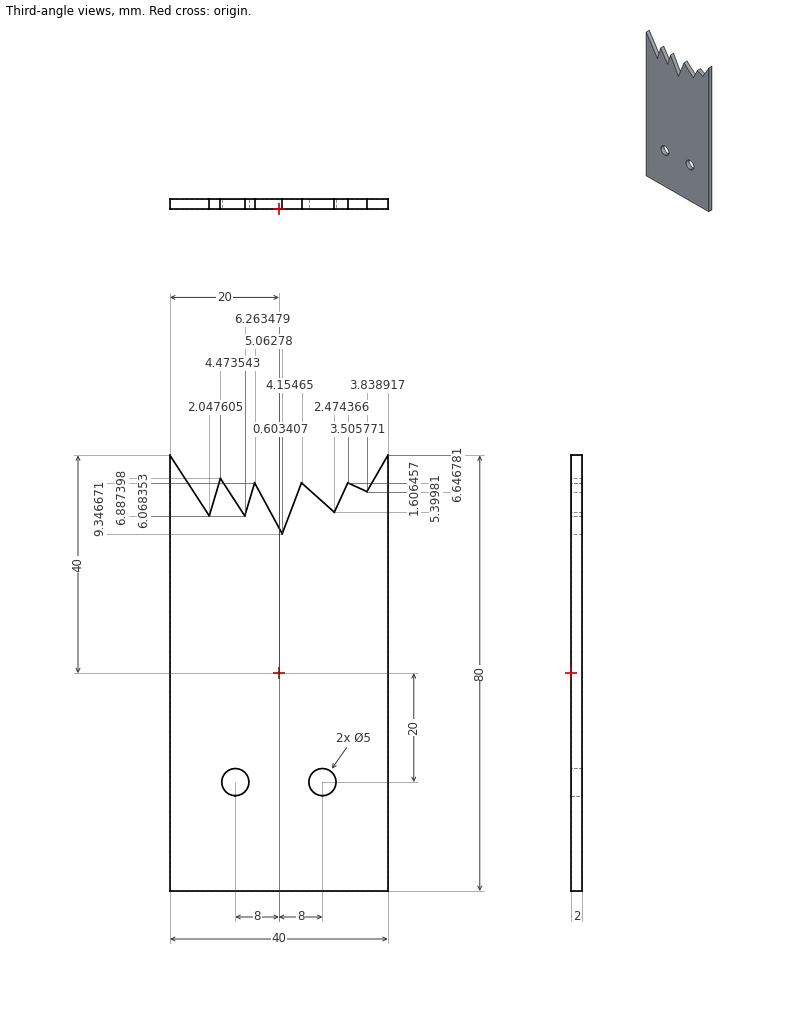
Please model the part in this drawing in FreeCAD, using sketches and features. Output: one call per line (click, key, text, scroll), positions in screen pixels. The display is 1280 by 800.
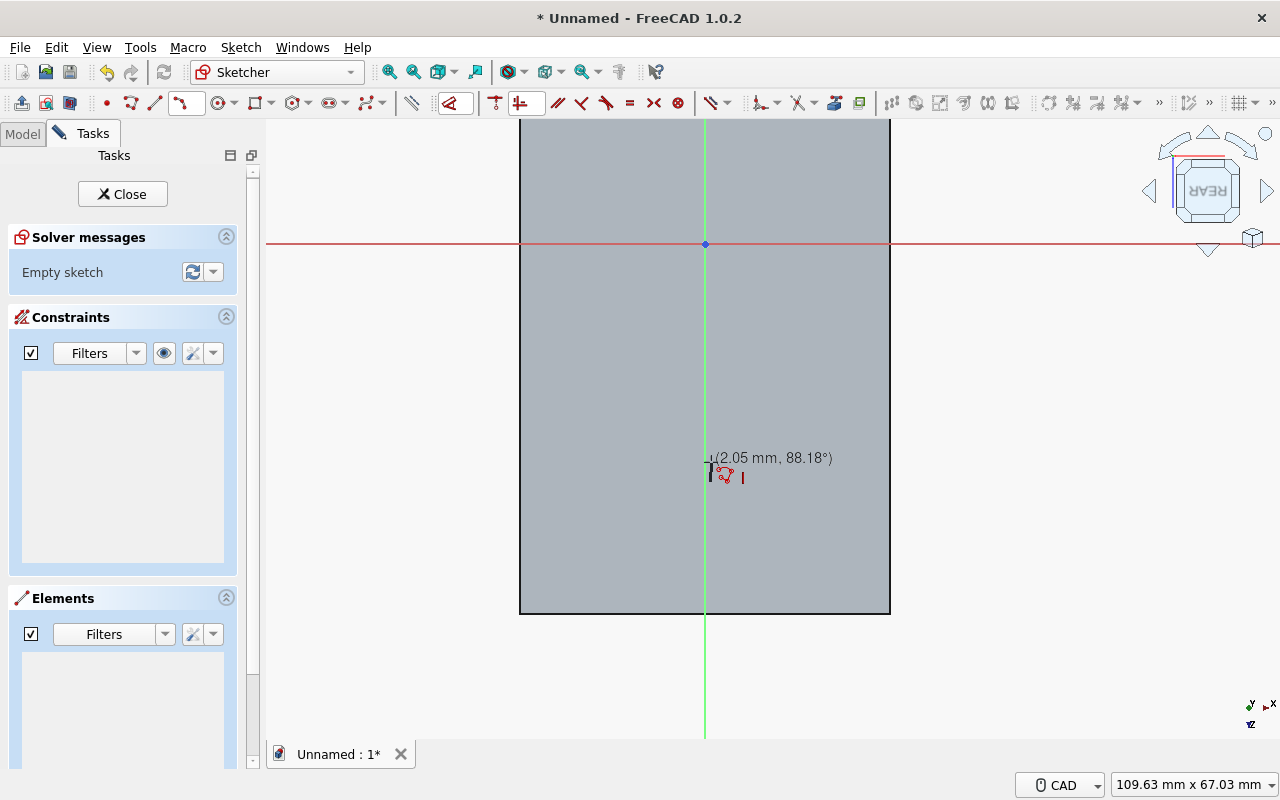
click(664, 568)
click(647, 512)
click(606, 575)
click(587, 512)
click(520, 614)
click(890, 614)
click(855, 553)
click(822, 568)
click(799, 518)
click(743, 568)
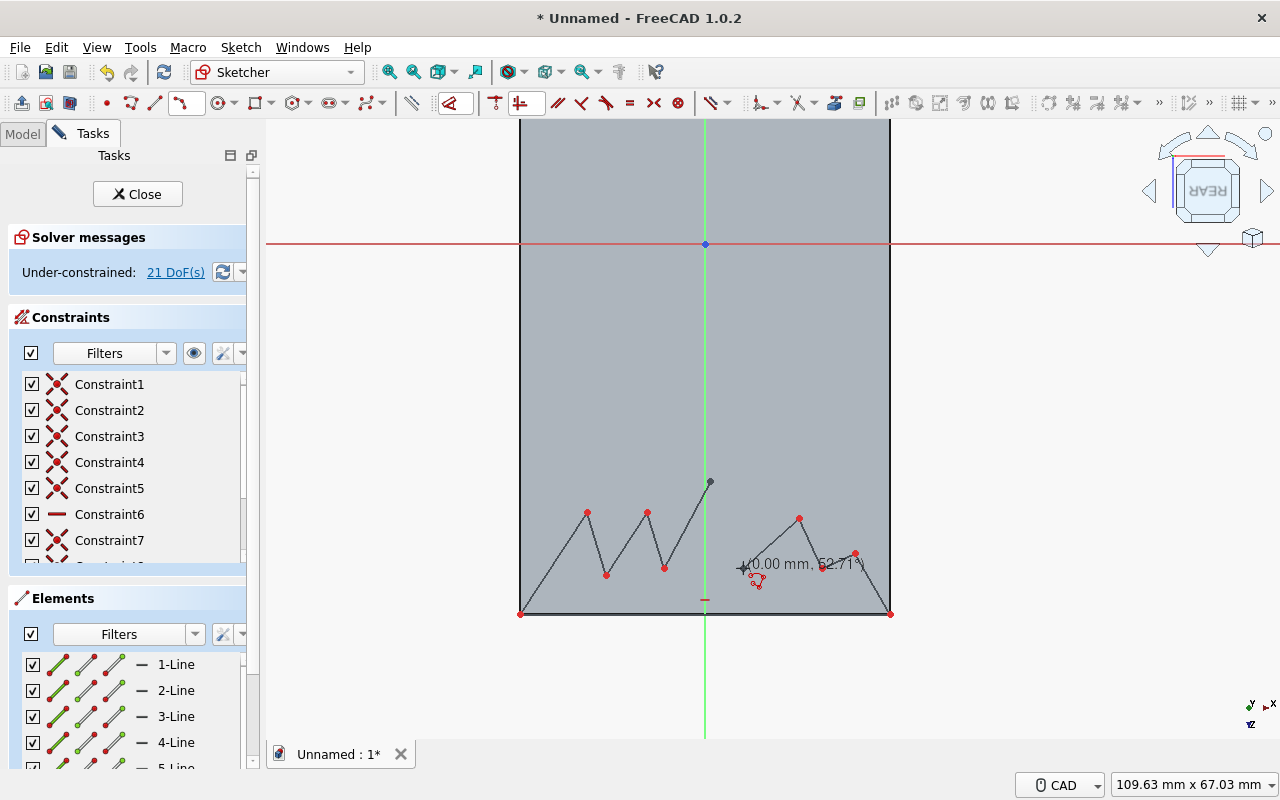
scroll(711, 481, up, 6)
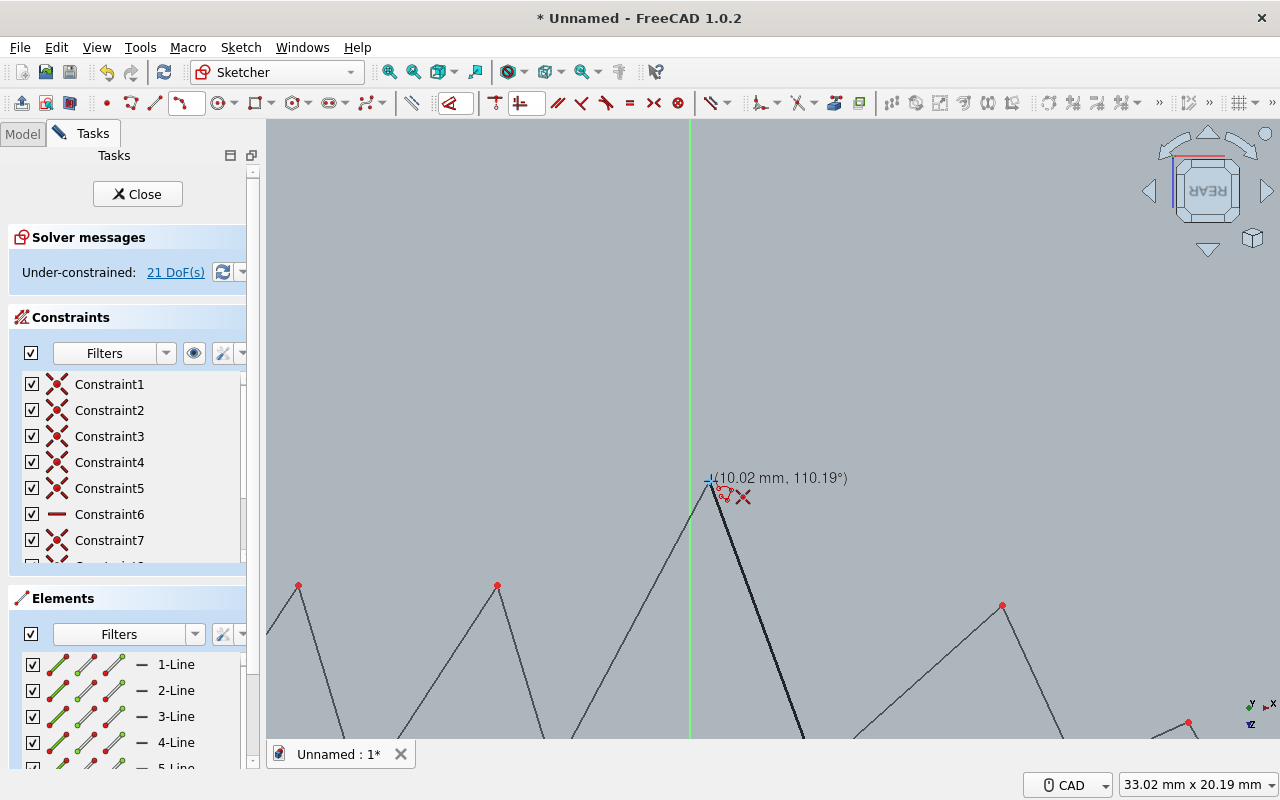
click(709, 482)
key(Escape)
key(Escape)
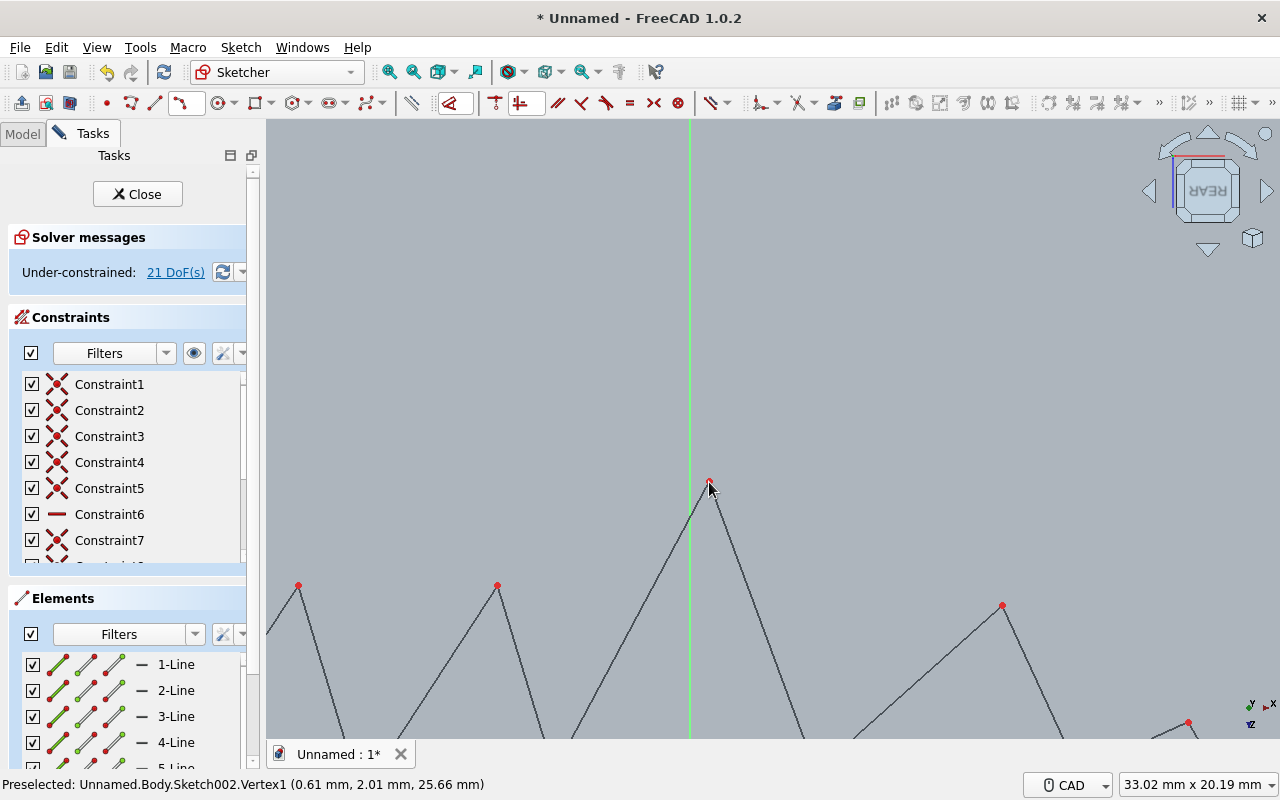
key(d)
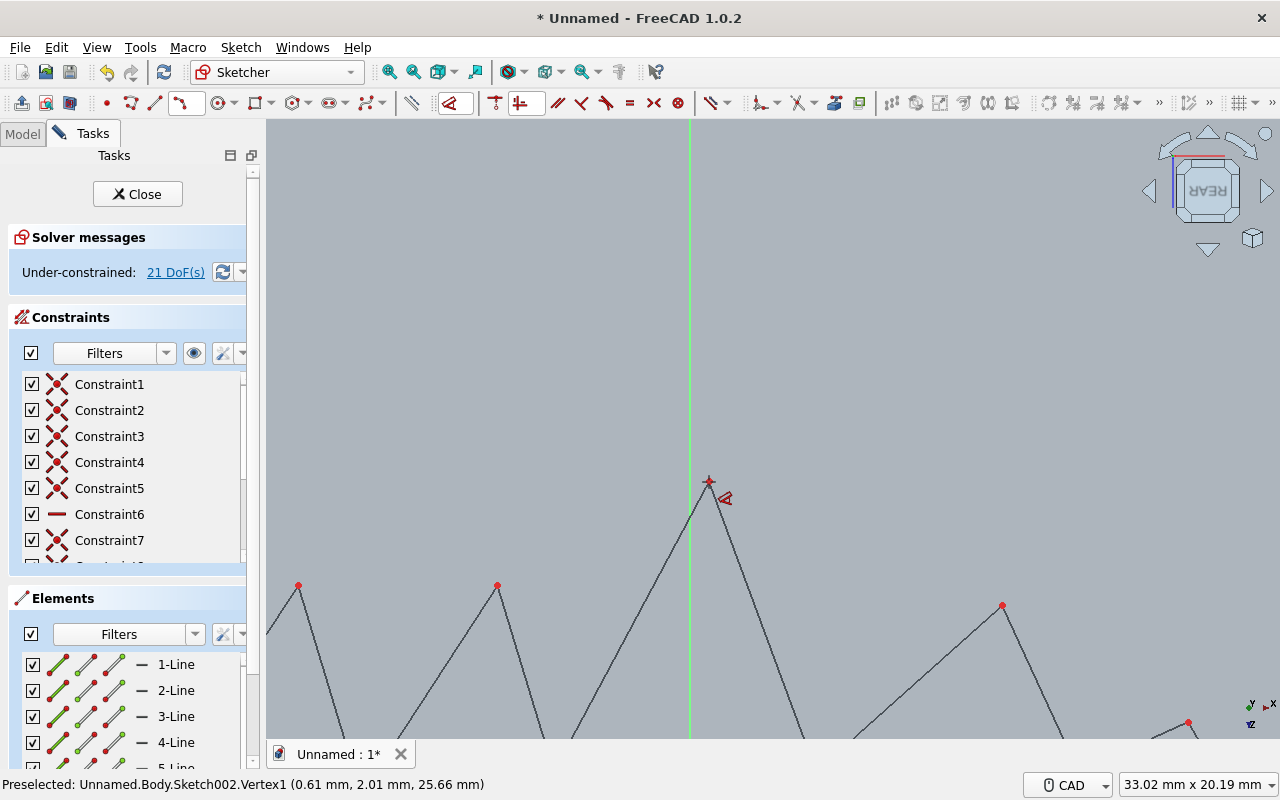
scroll(711, 481, down, 6)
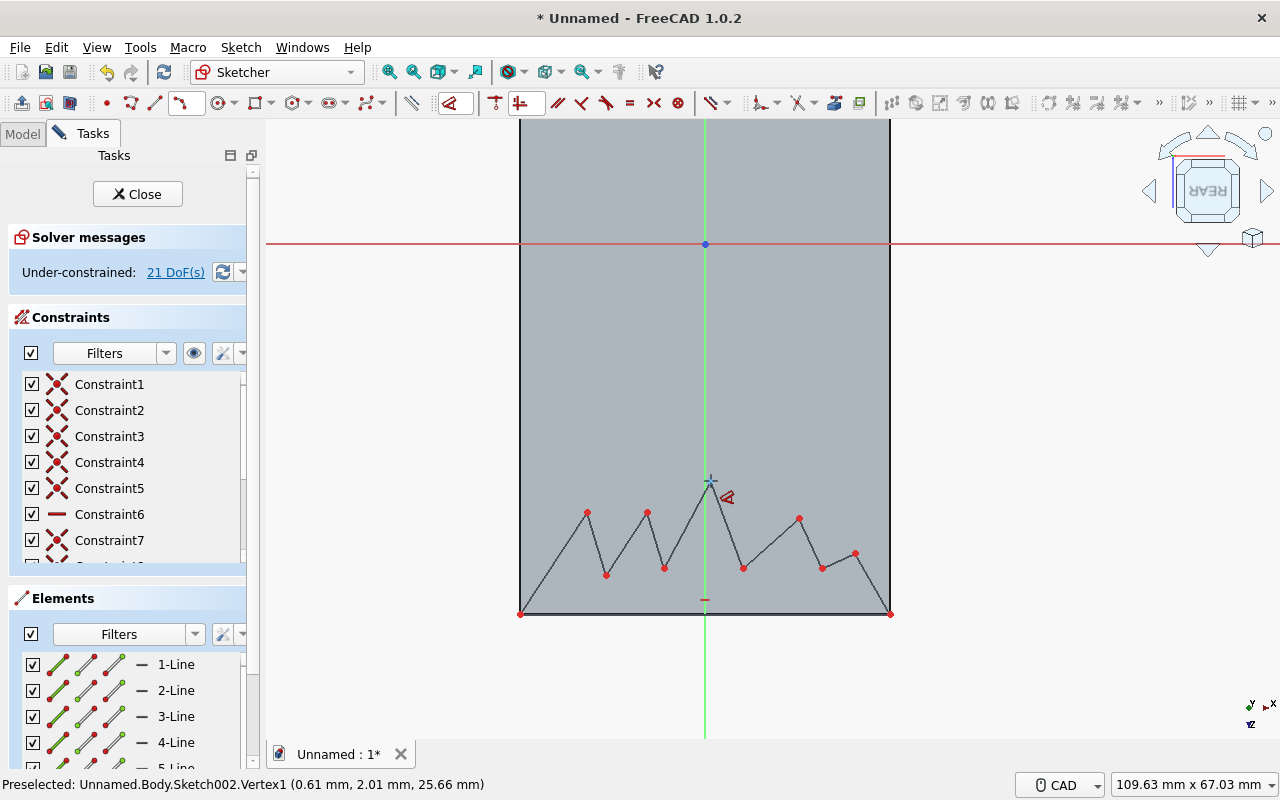
click(631, 615)
click(620, 649)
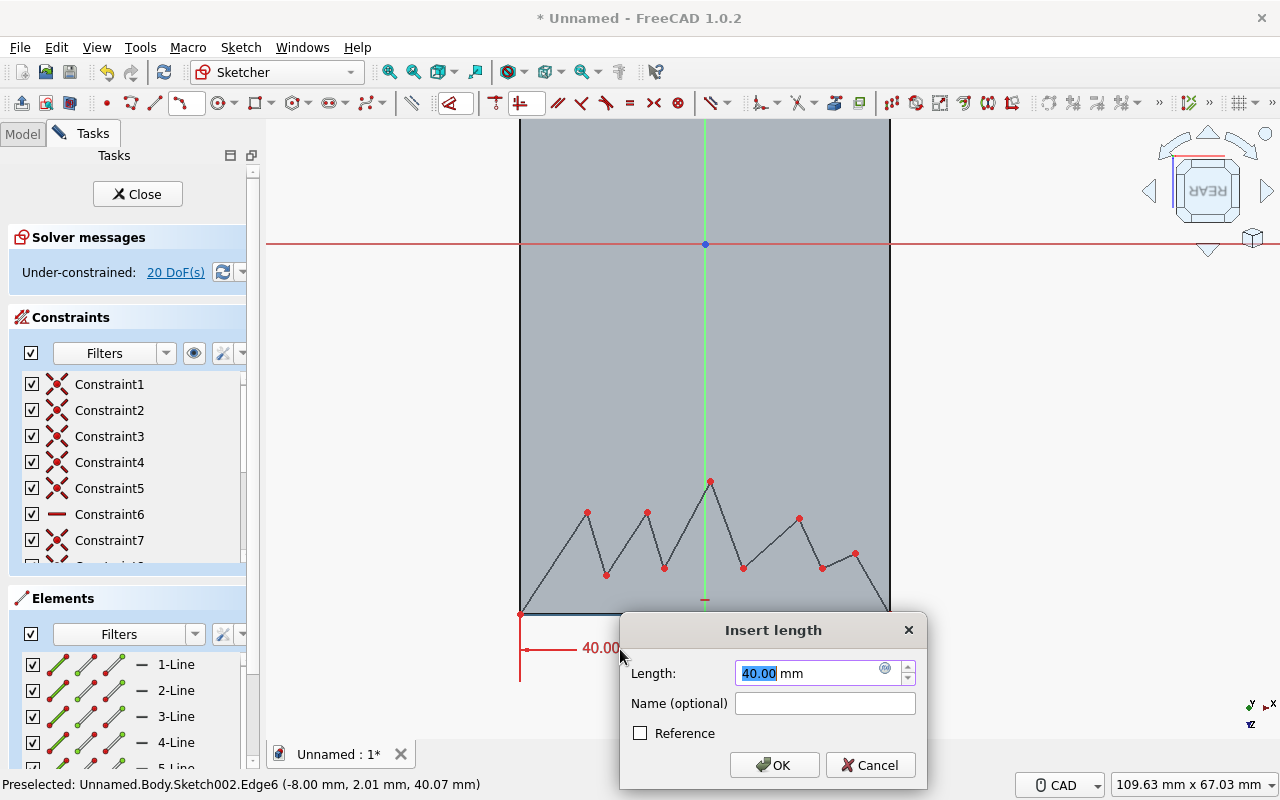
text(40)
key(Return)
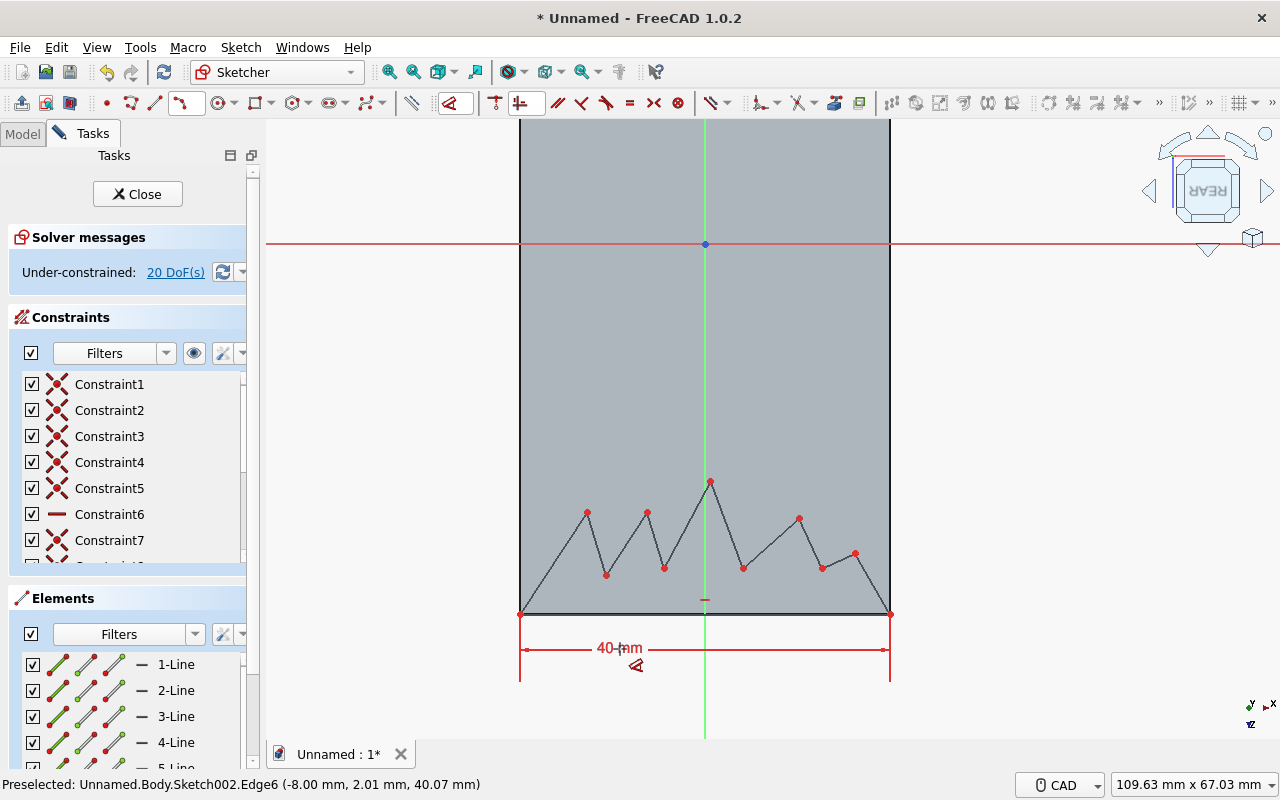
click(520, 615)
click(548, 649)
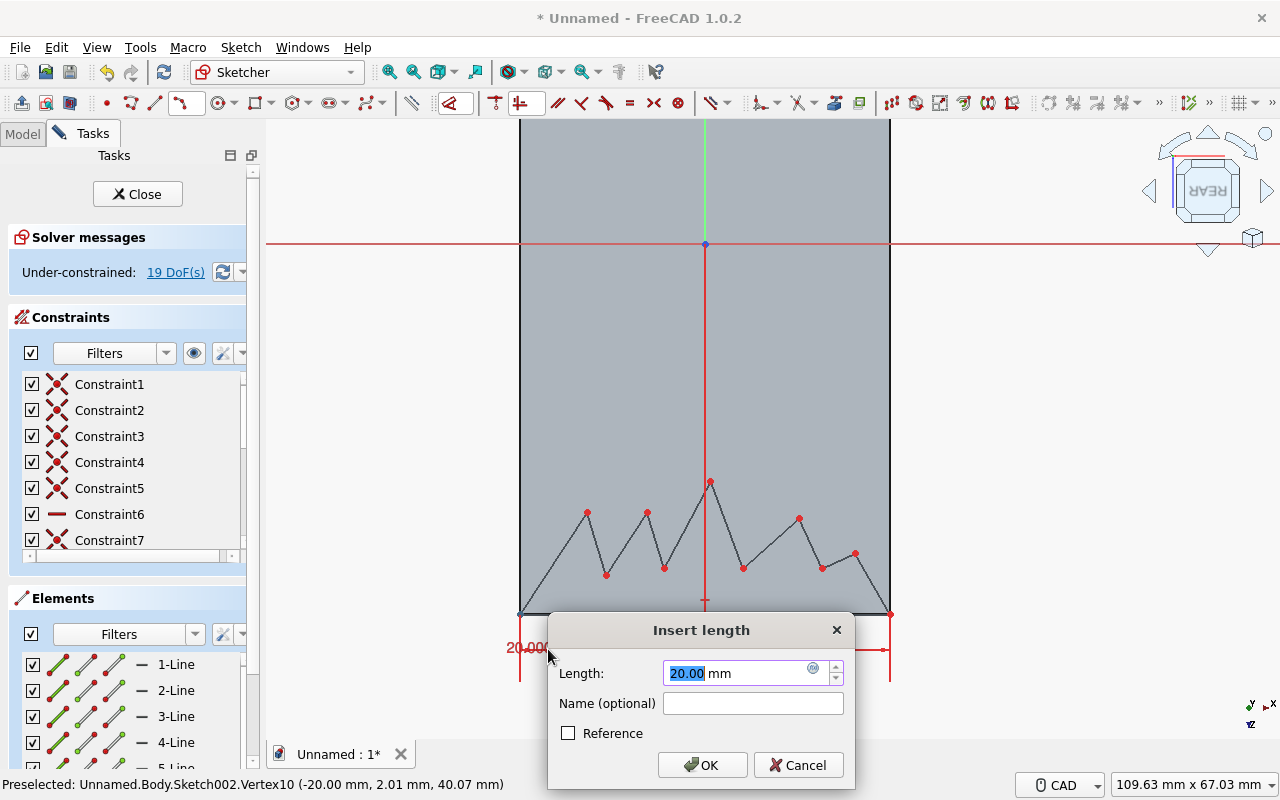
text(20)
key(Return)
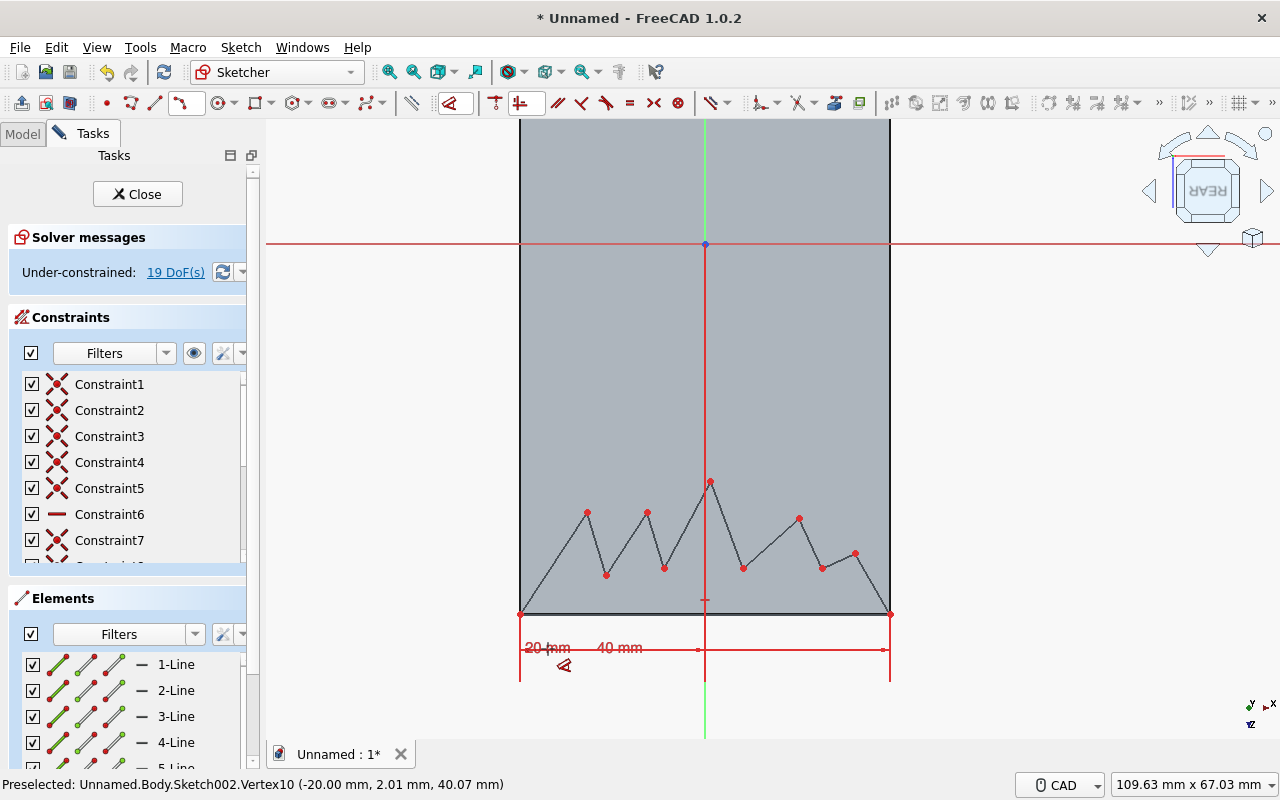
click(520, 615)
click(486, 430)